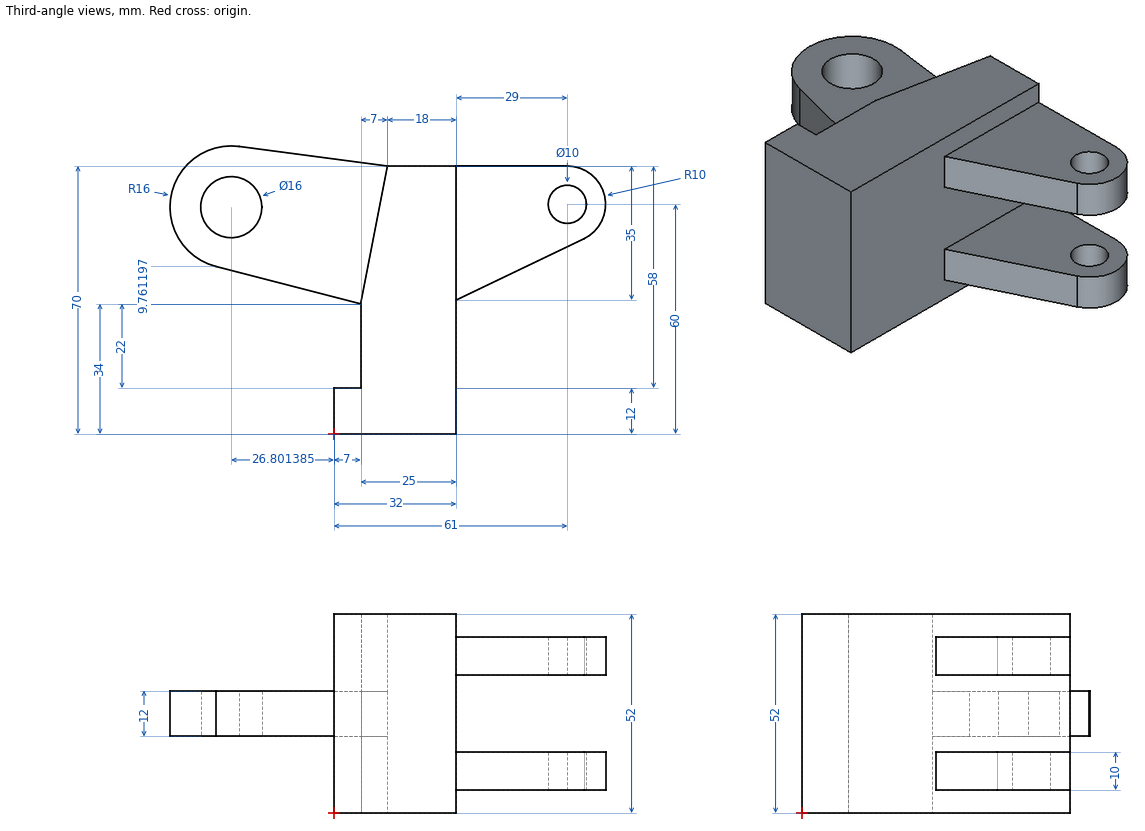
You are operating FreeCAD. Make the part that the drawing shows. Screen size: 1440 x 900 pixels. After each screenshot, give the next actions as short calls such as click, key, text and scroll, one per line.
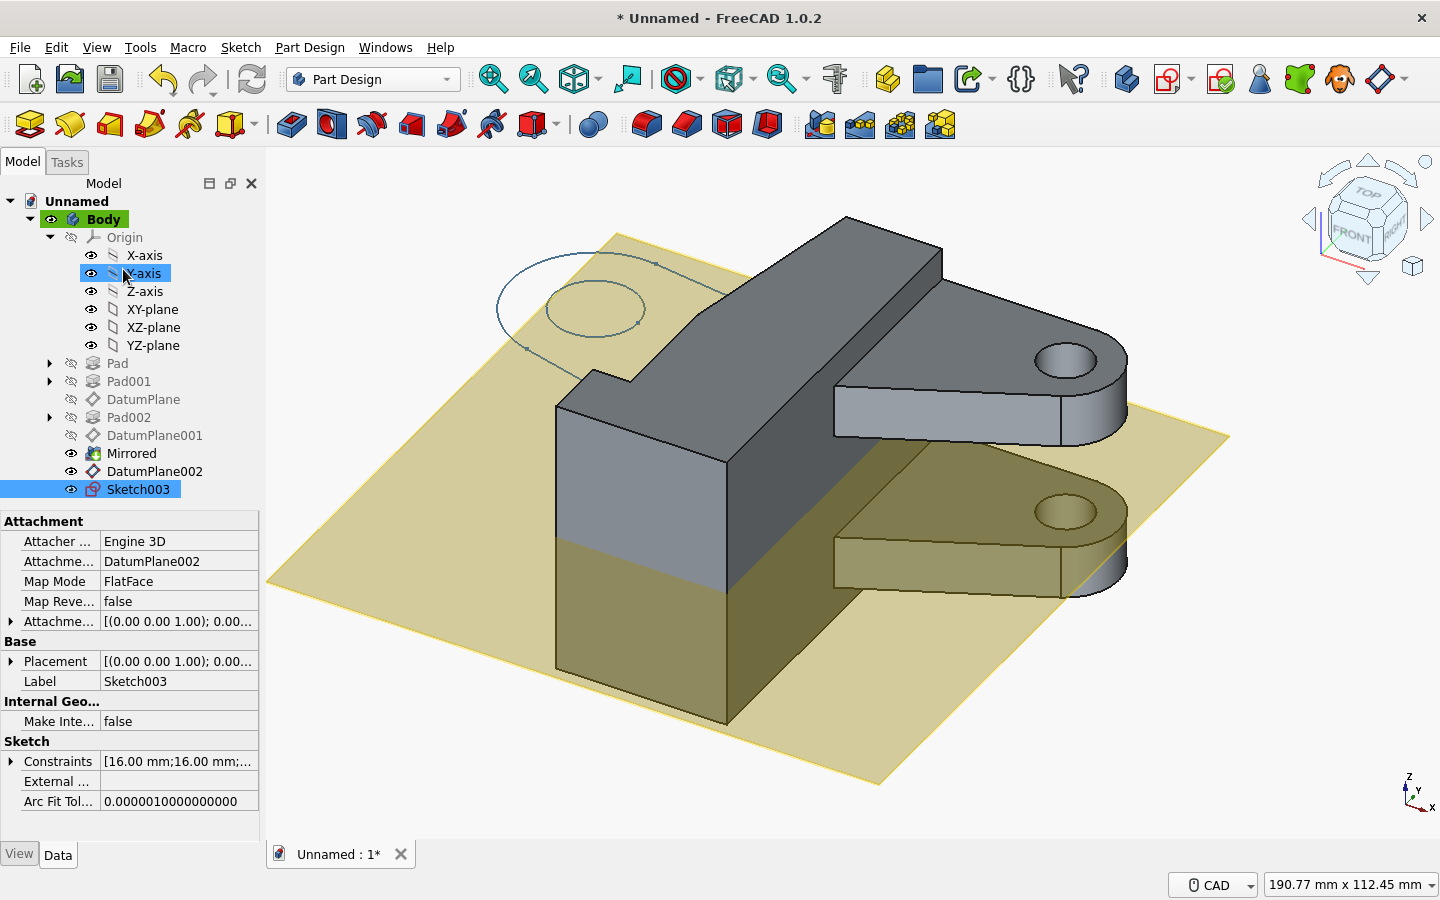
click(30, 124)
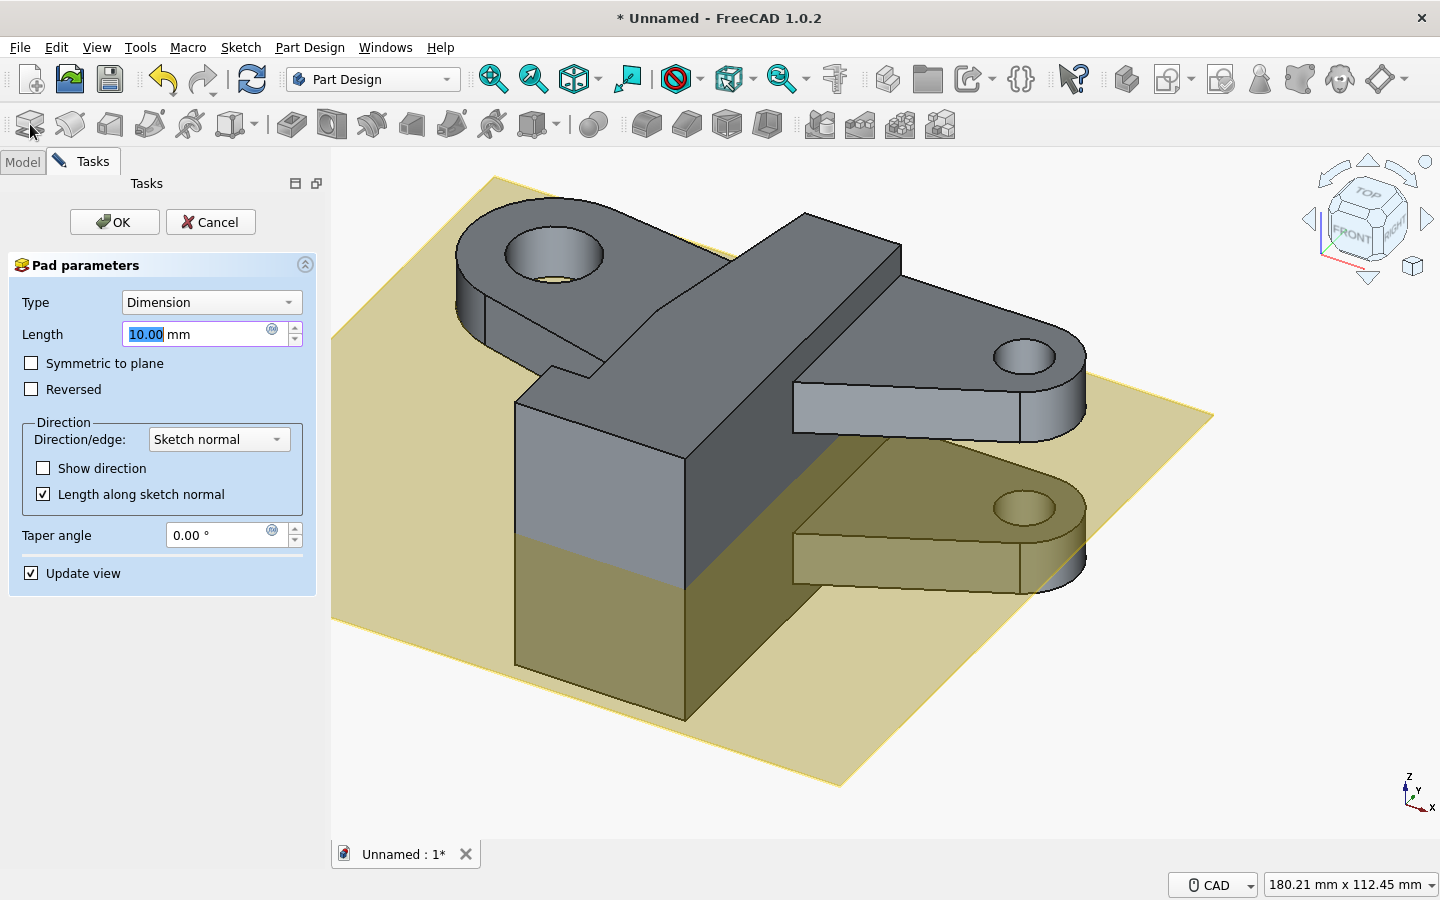
text(12)
key(Tab)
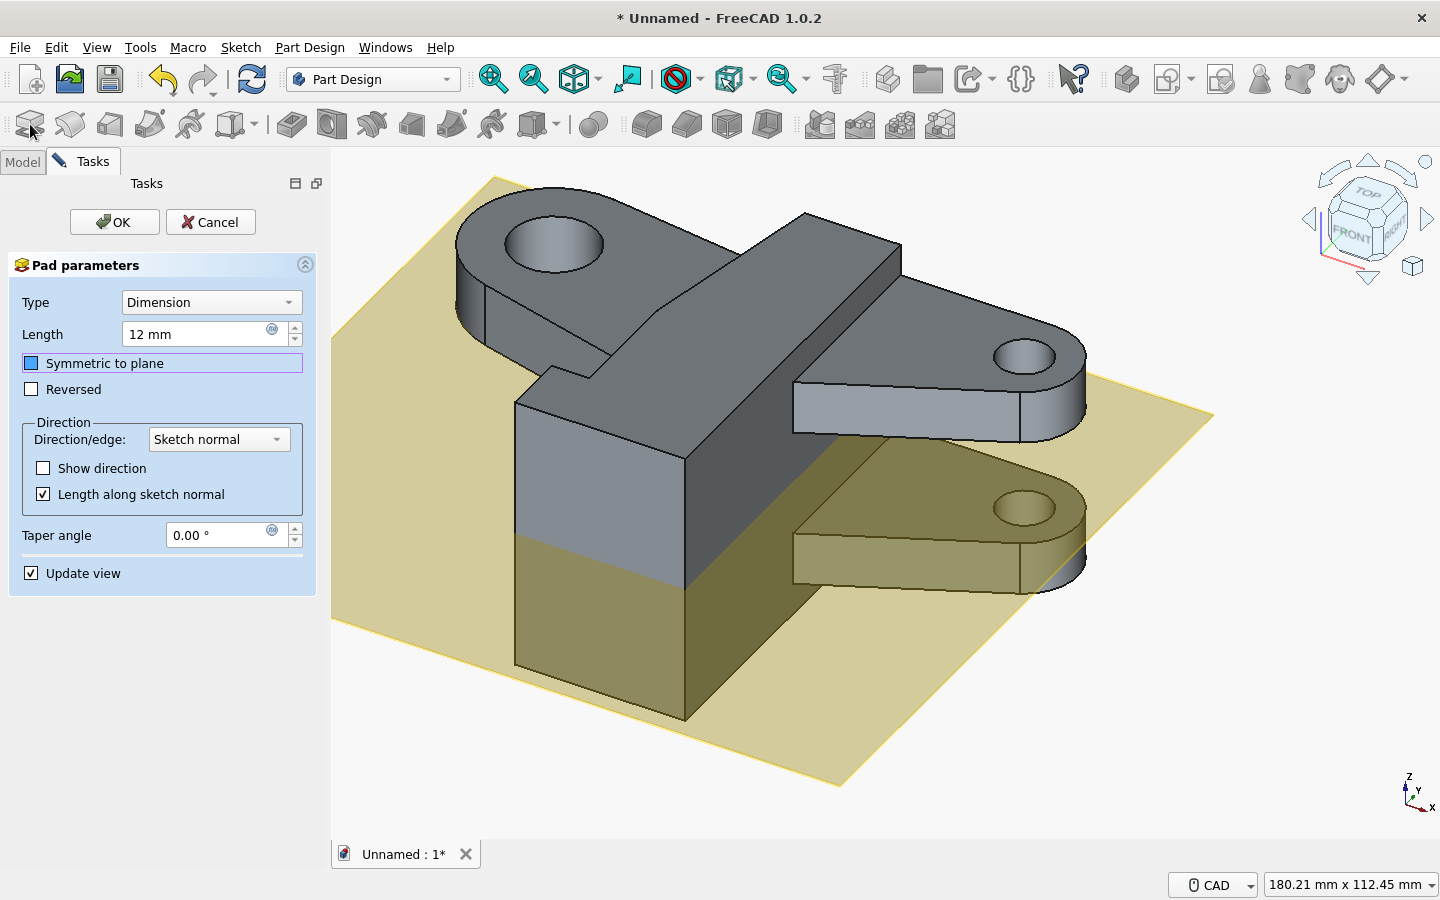
click(30, 363)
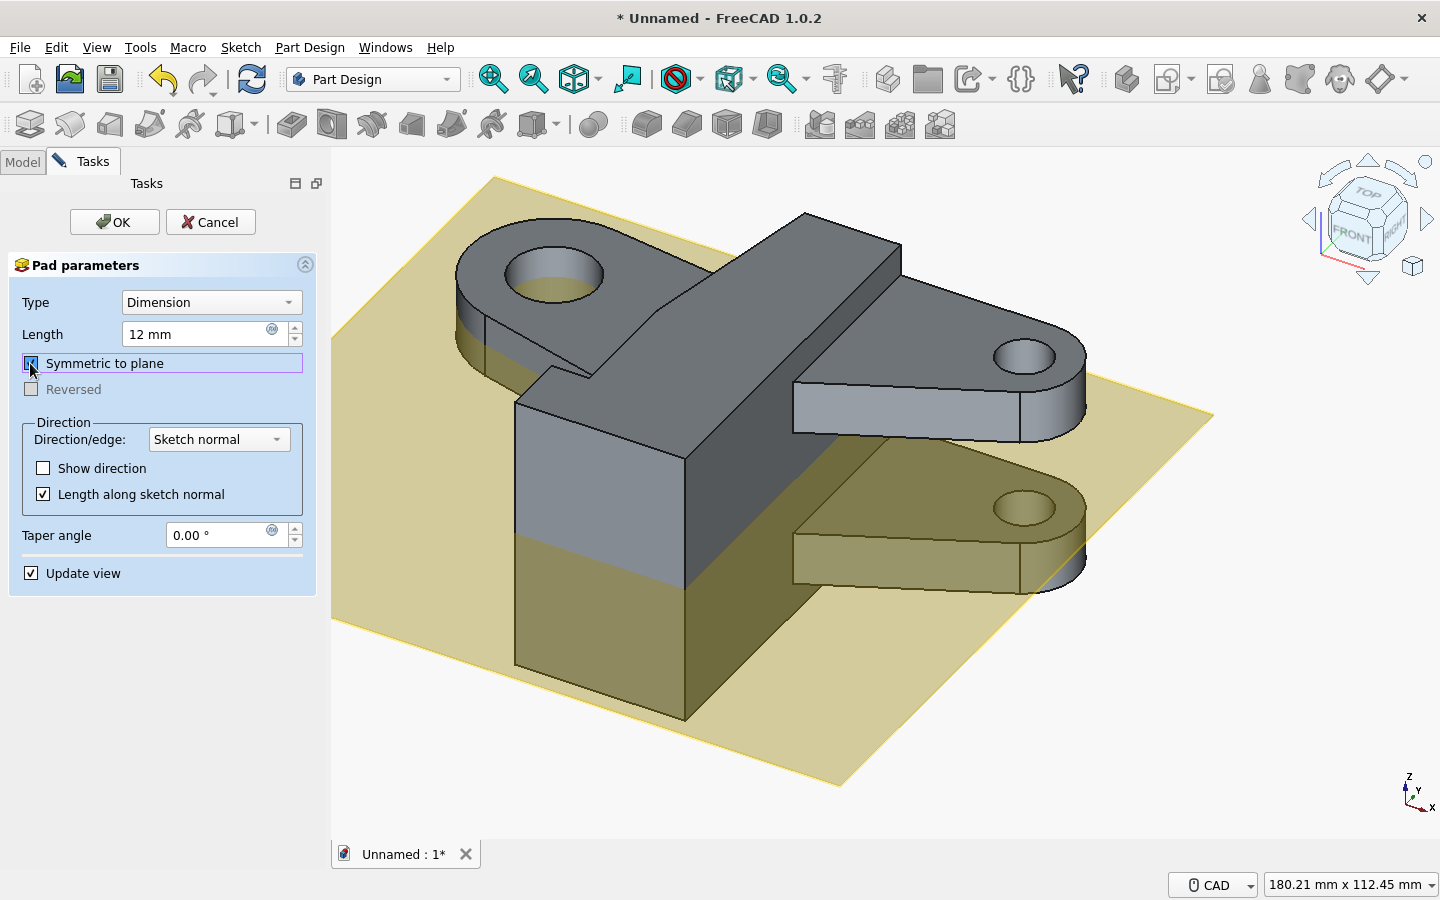
click(115, 222)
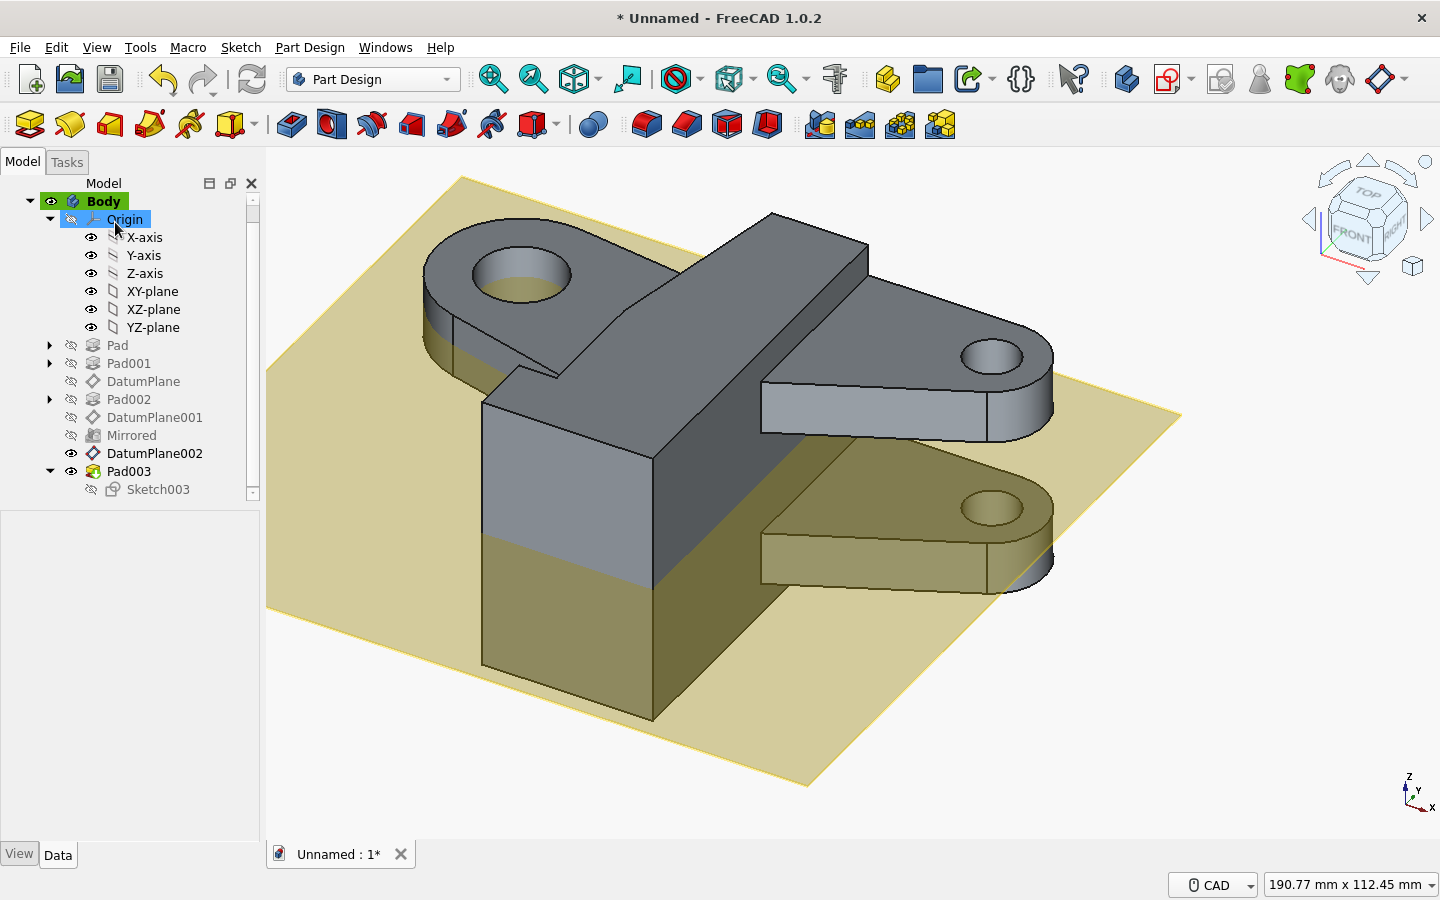
click(116, 453)
key(space)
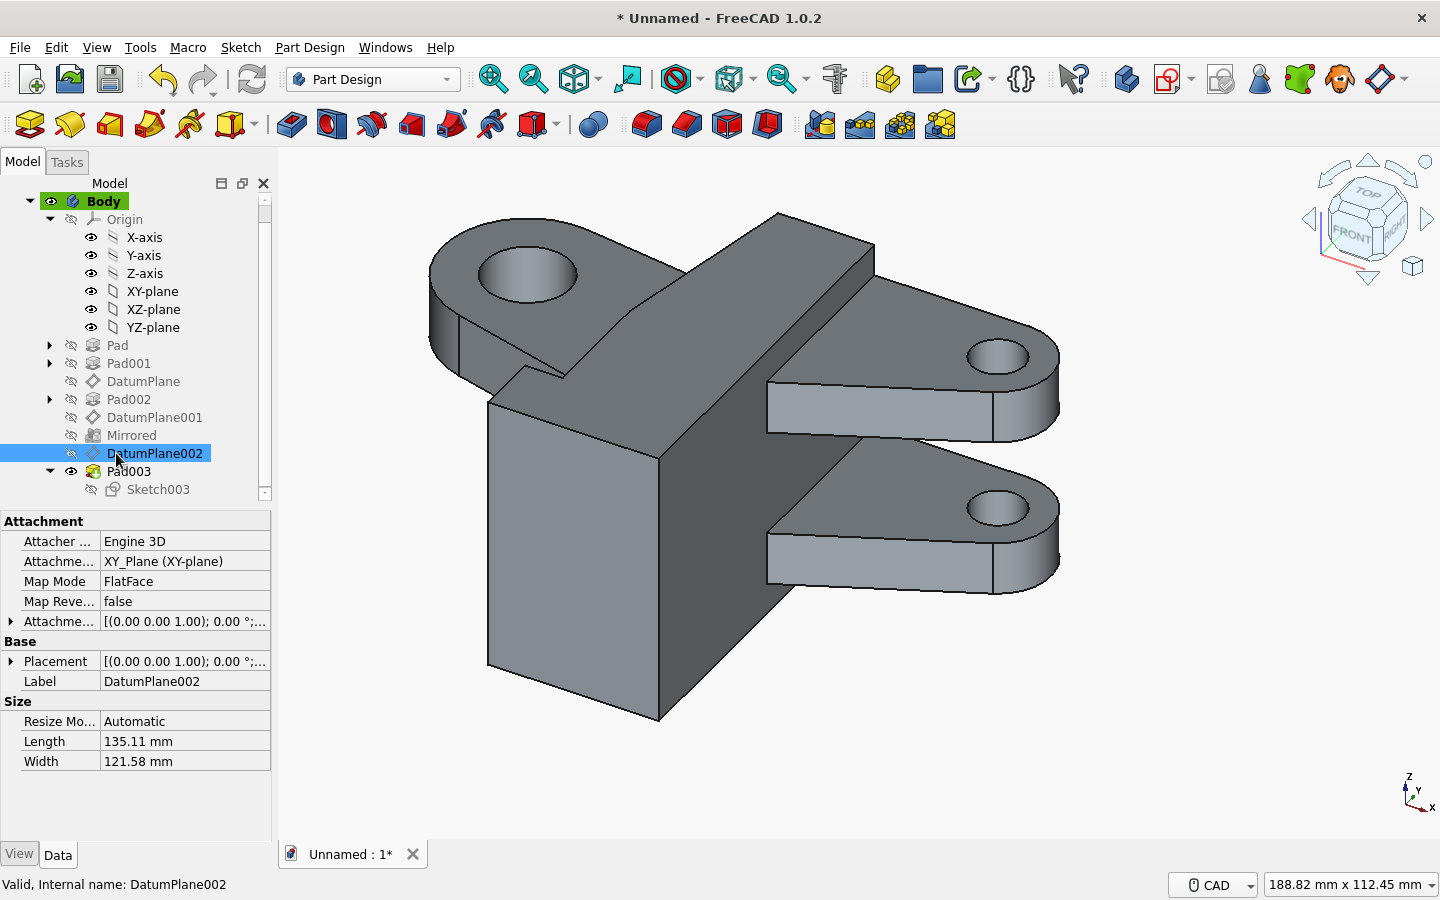
key(0)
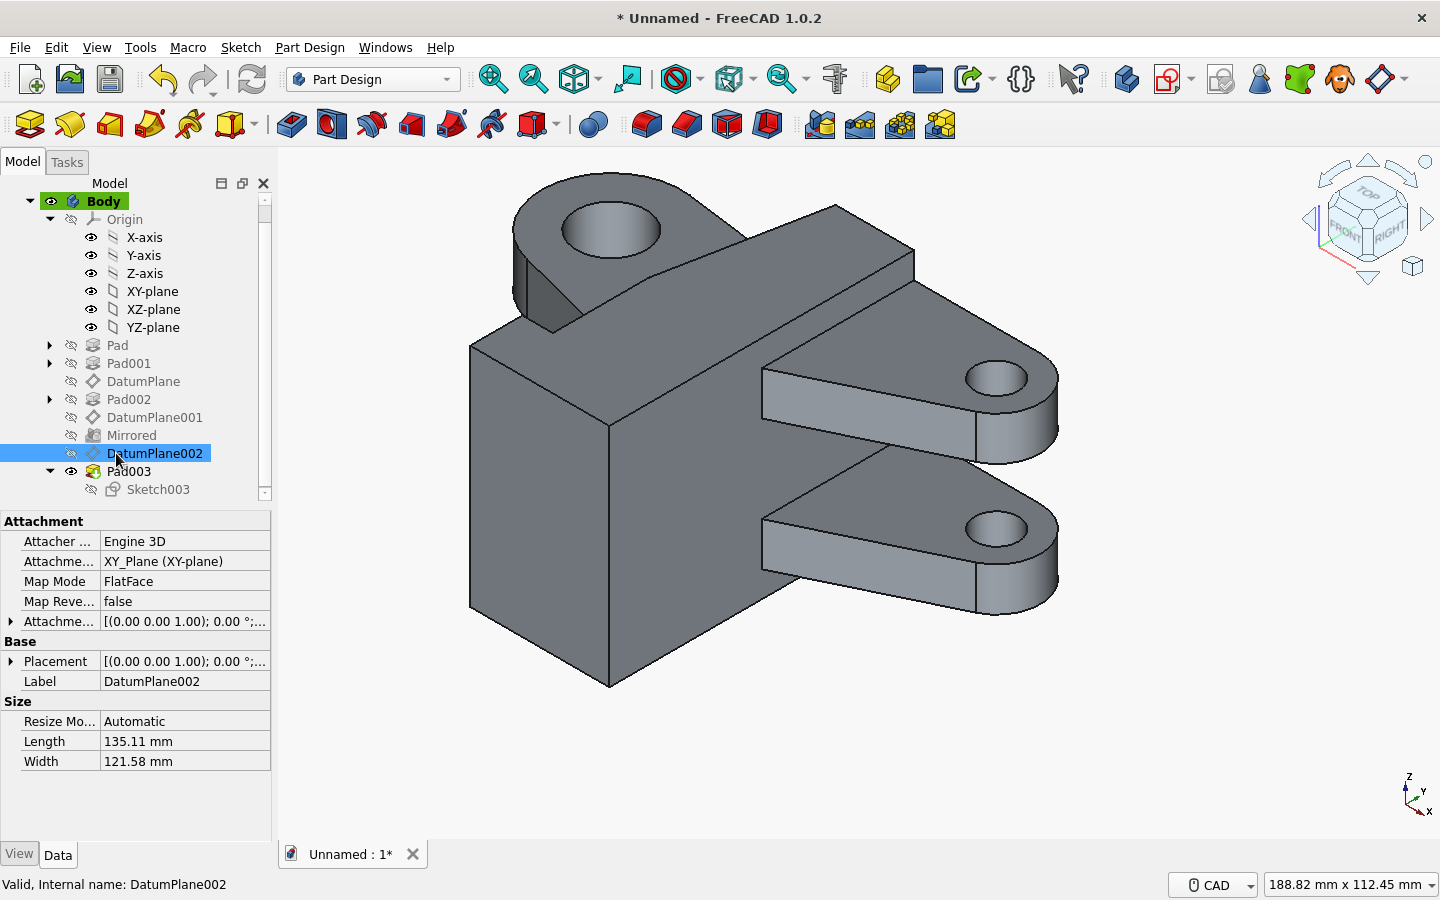
click(494, 80)